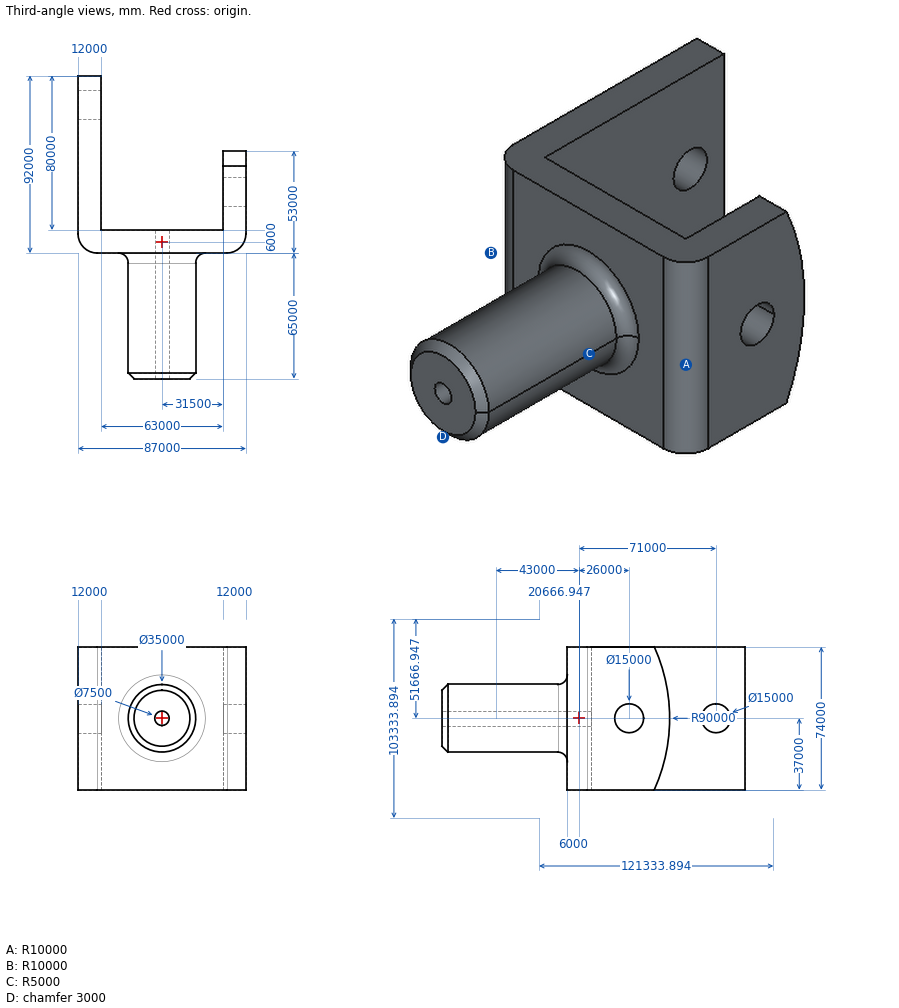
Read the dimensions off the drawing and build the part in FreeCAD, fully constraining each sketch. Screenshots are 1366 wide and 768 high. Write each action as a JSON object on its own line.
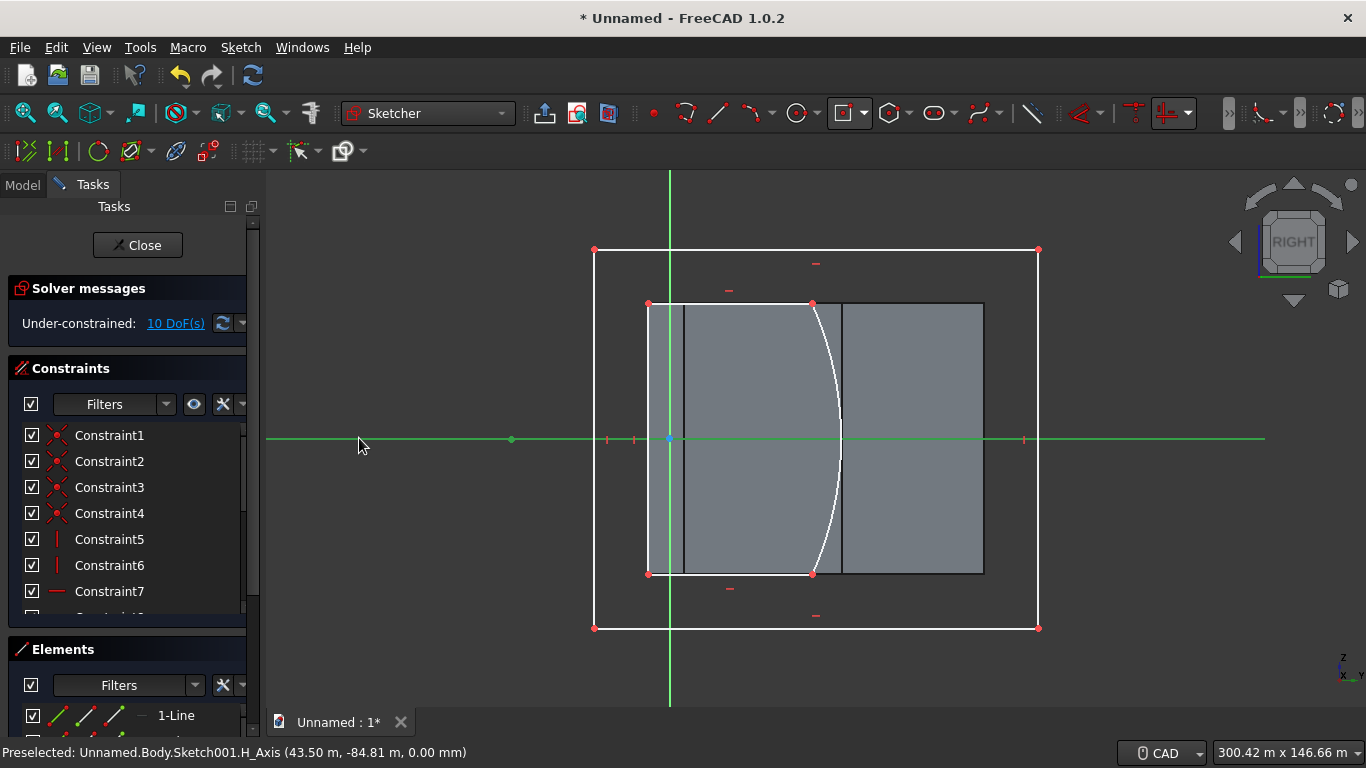
{"action": "left_click", "coordinate": [1134, 114]}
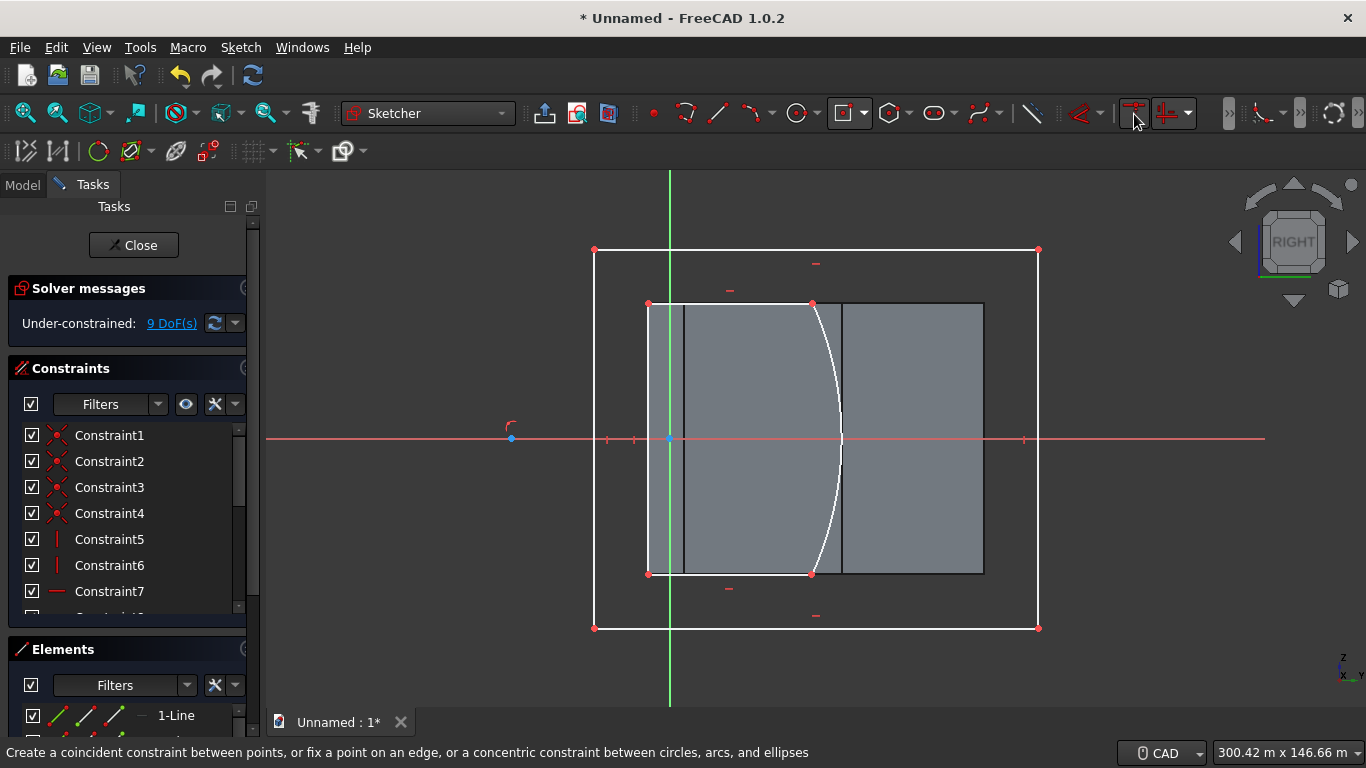
{"action": "left_click", "coordinate": [1080, 114]}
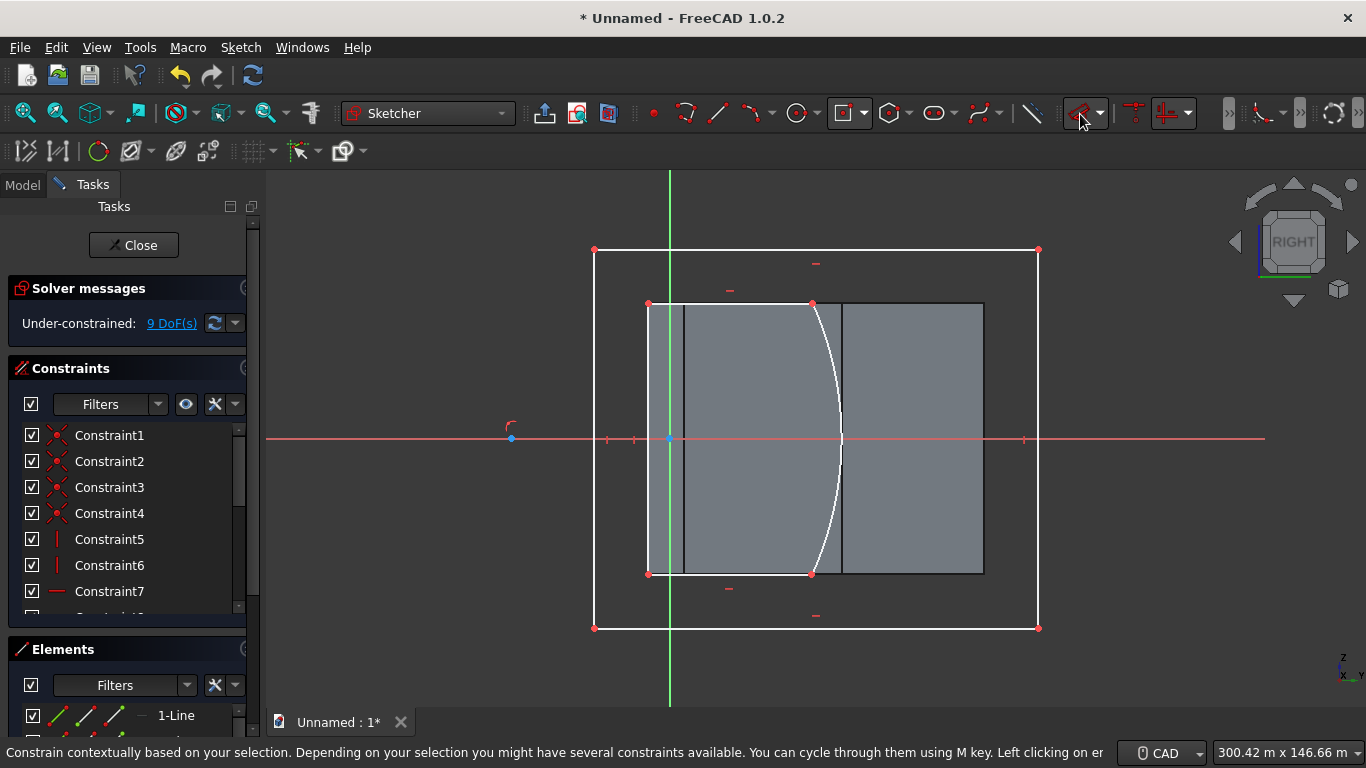
{"action": "left_click", "coordinate": [837, 495]}
{"action": "left_click", "coordinate": [869, 500]}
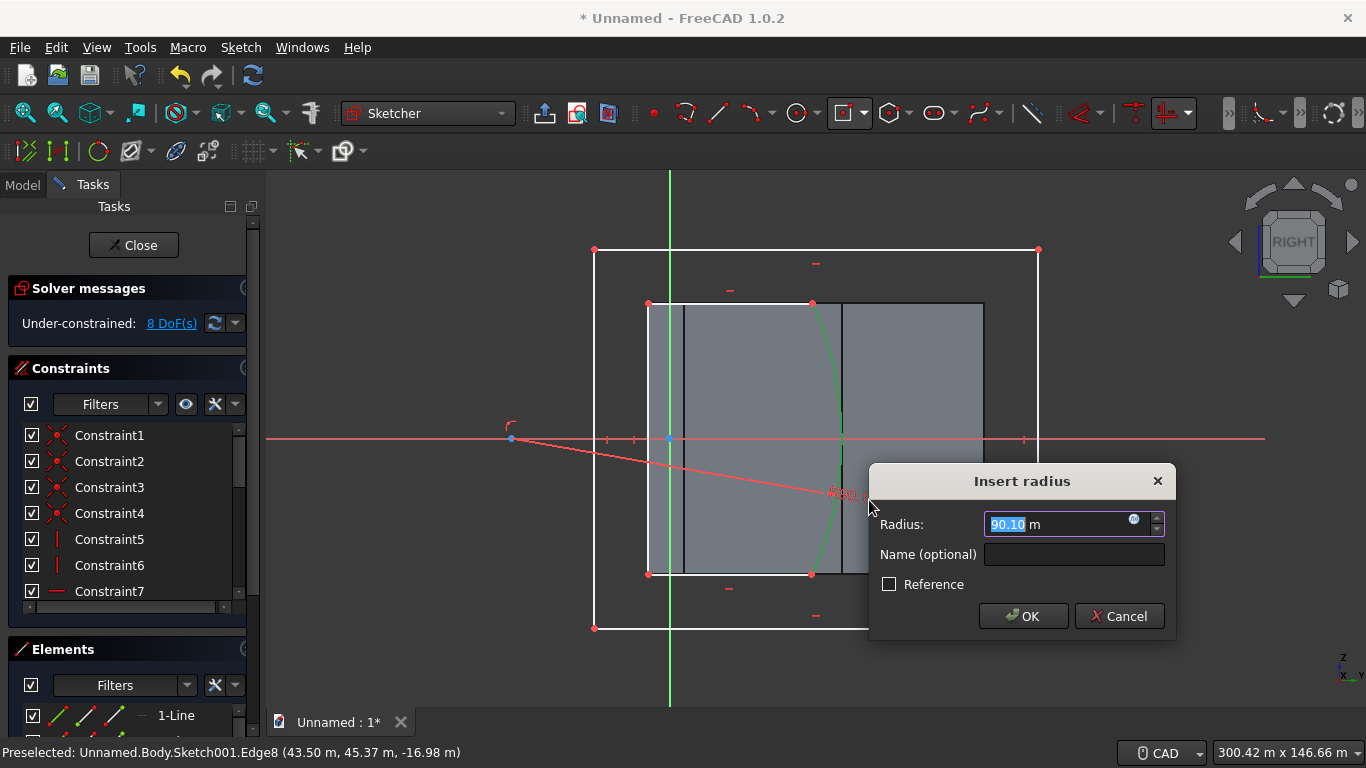
{"action": "key", "text": "ctrl+a"}
{"action": "type", "text": "90000 mm"}
{"action": "key", "text": "Return"}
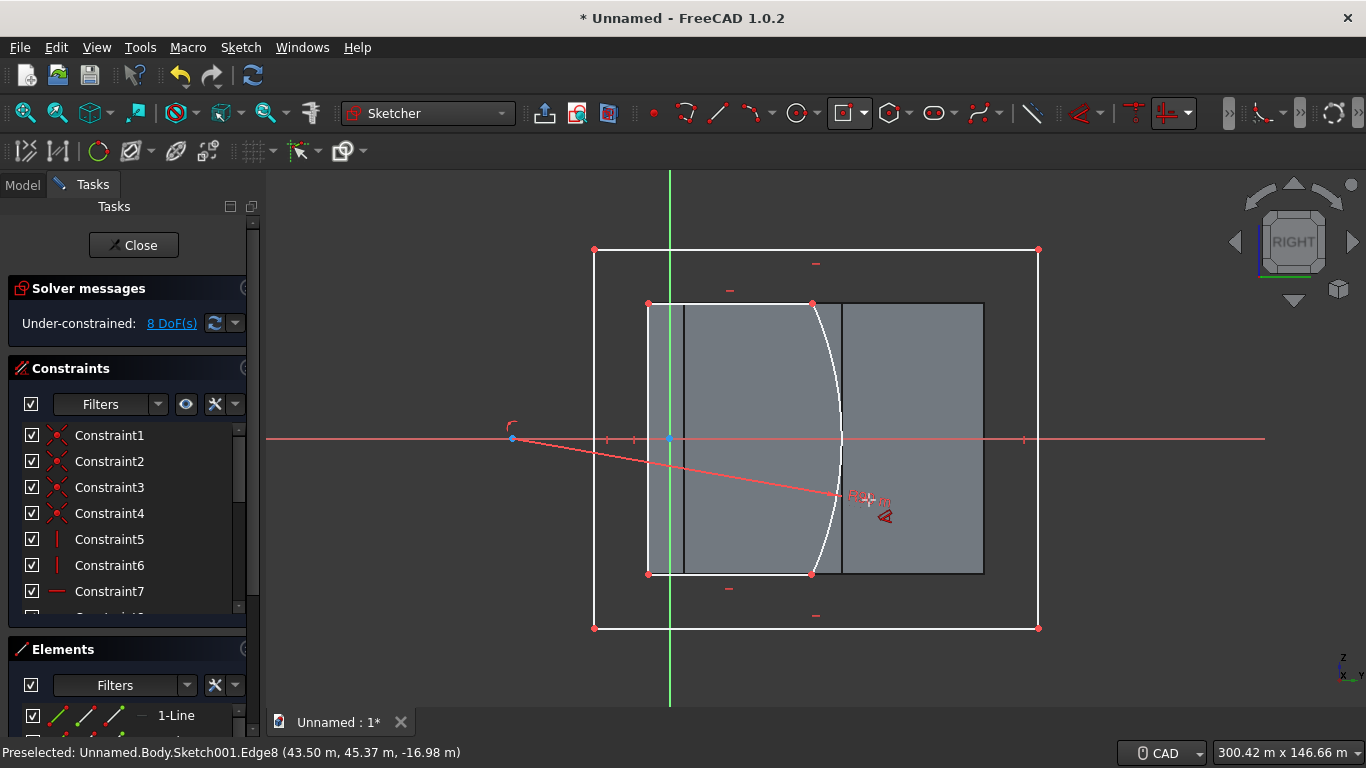
{"action": "left_click", "coordinate": [648, 494]}
{"action": "left_click", "coordinate": [614, 377]}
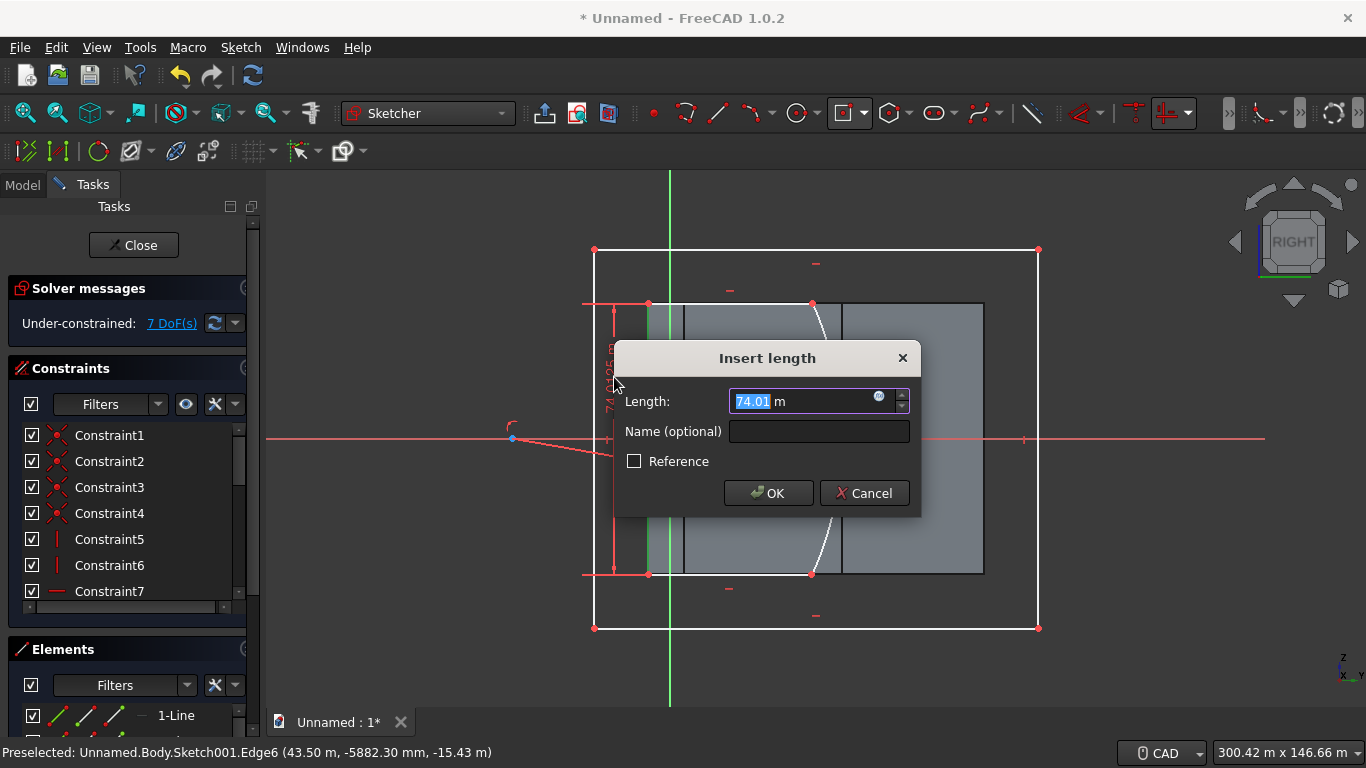
{"action": "key", "text": "ctrl+a"}
{"action": "type", "text": "74000 mm"}
{"action": "key", "text": "Return"}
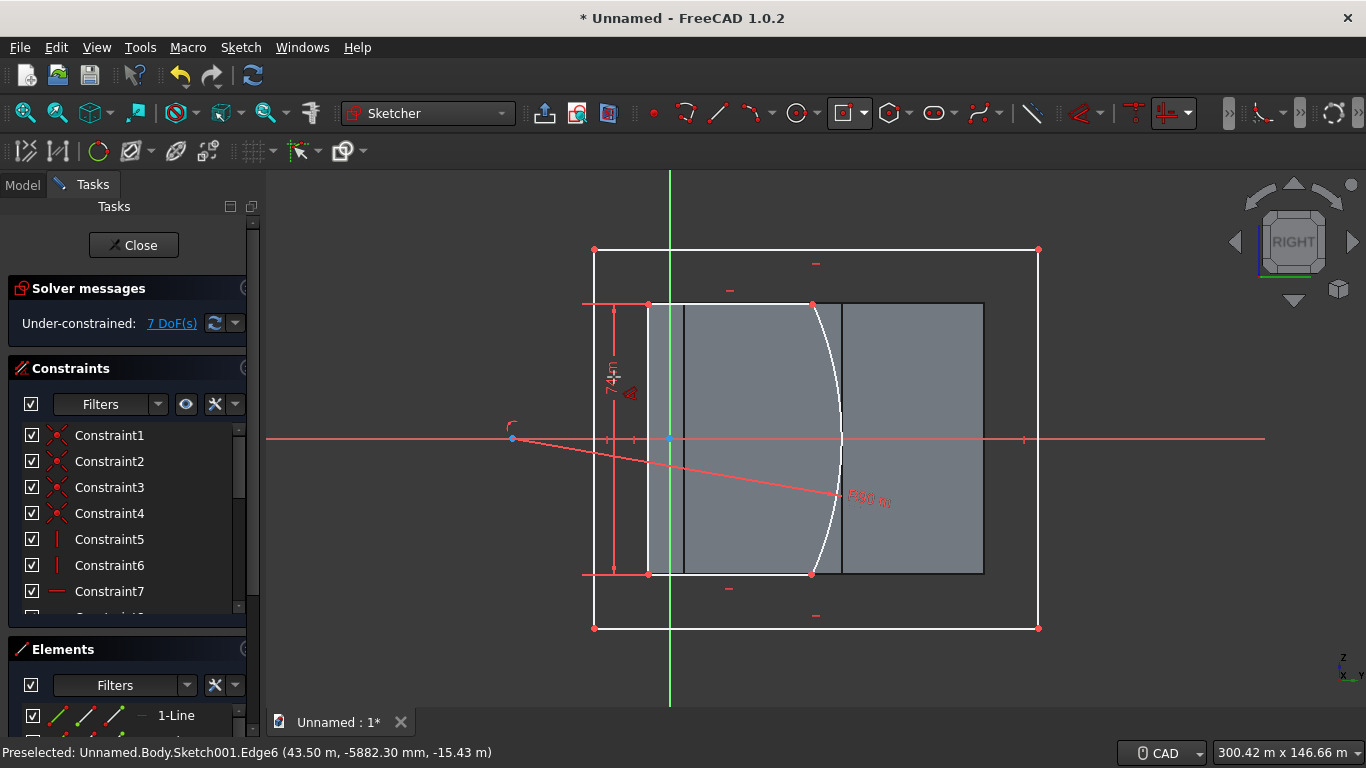
{"action": "scroll", "coordinate": [648, 575], "scroll_direction": "up", "scroll_amount": 3}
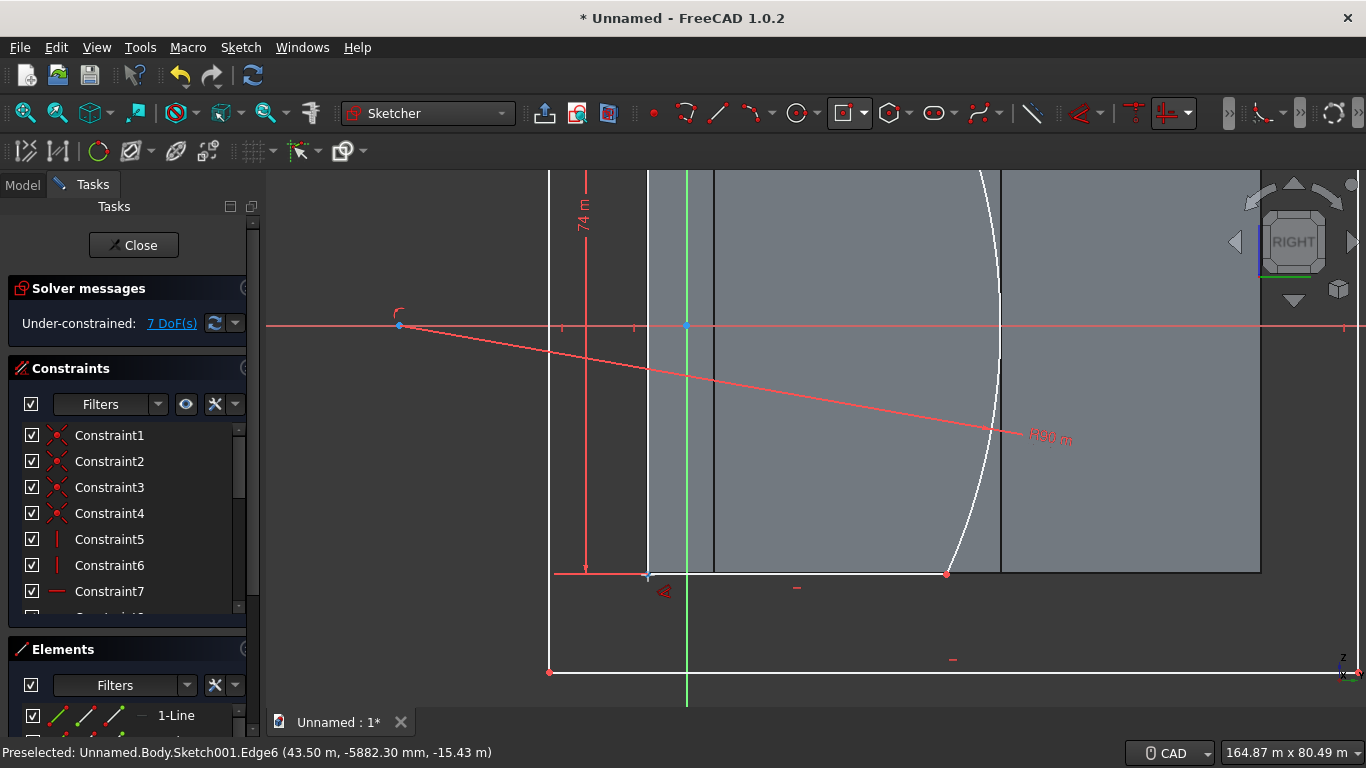
{"action": "left_click", "coordinate": [648, 574]}
{"action": "left_click", "coordinate": [667, 608]}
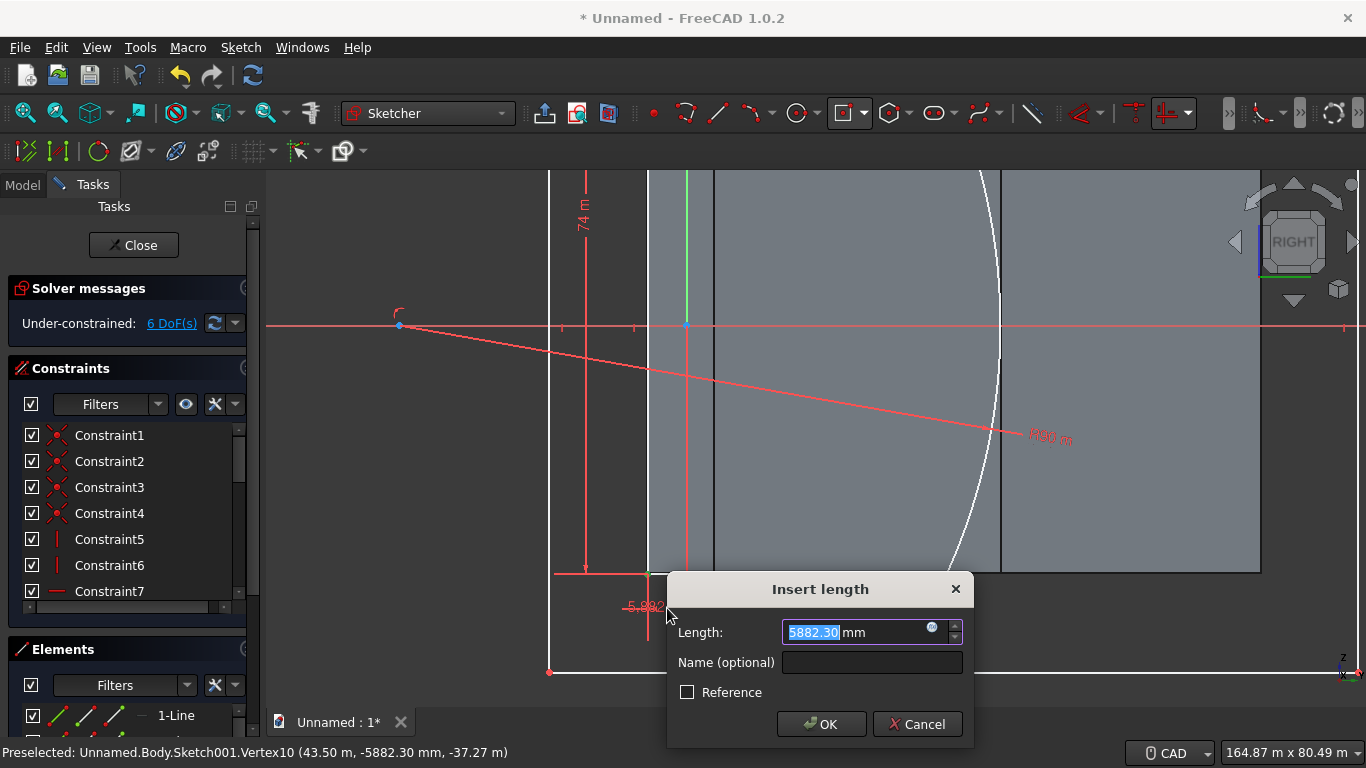
{"action": "type", "text": "6000"}
{"action": "key", "text": "Return"}